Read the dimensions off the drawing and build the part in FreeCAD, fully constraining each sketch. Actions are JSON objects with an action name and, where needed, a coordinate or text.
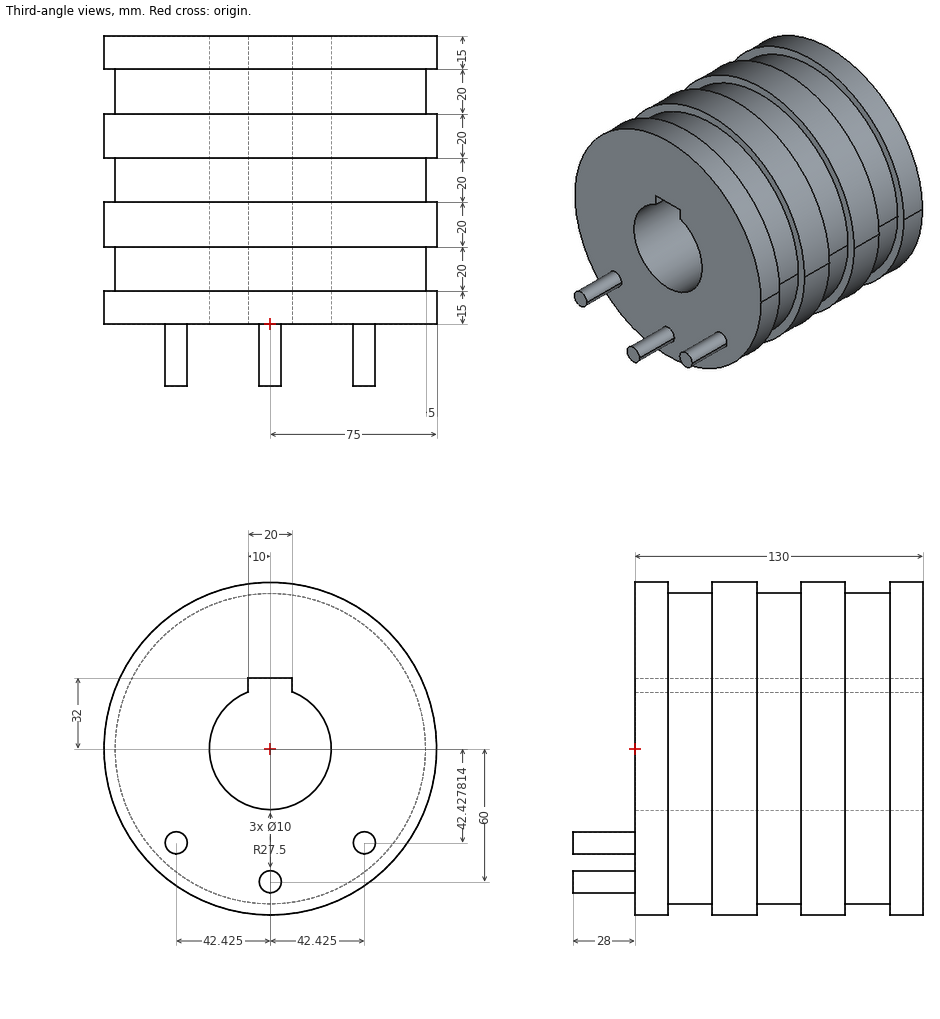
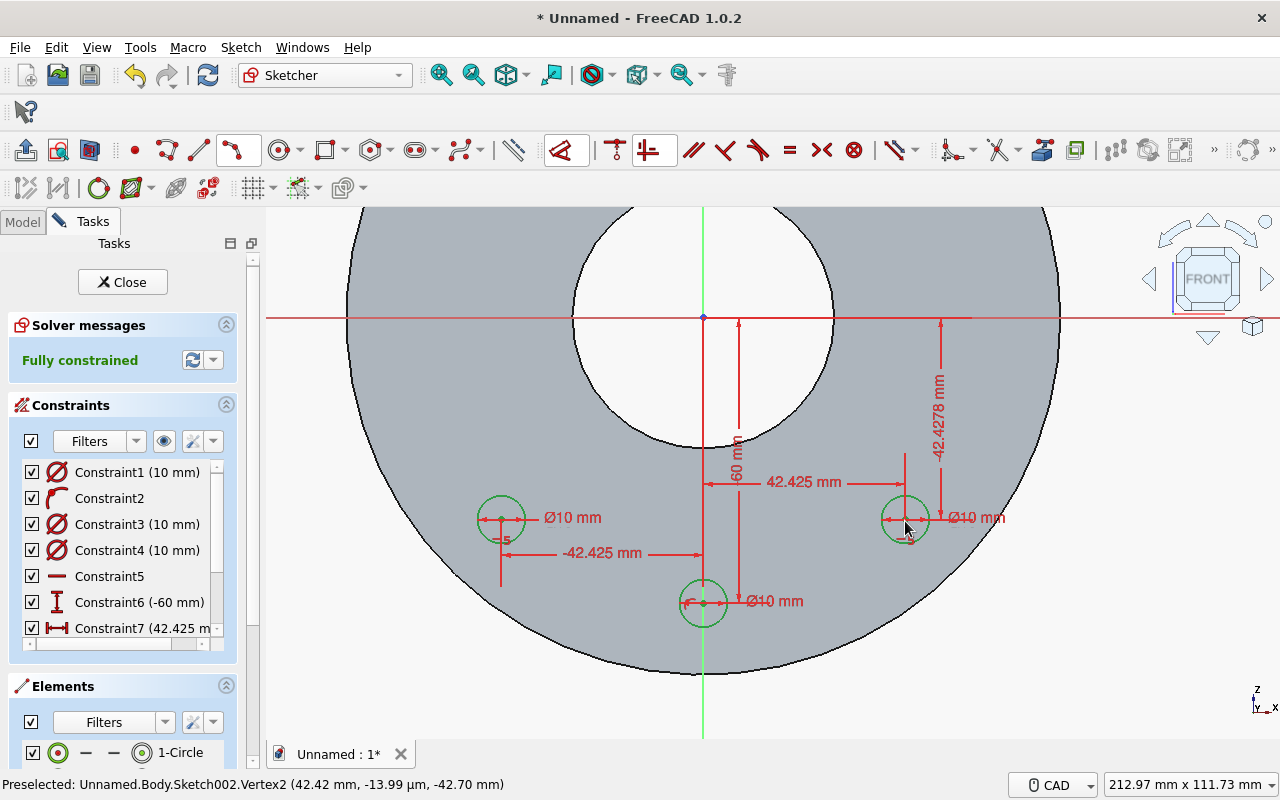
{"action": "left_click", "coordinate": [123, 282]}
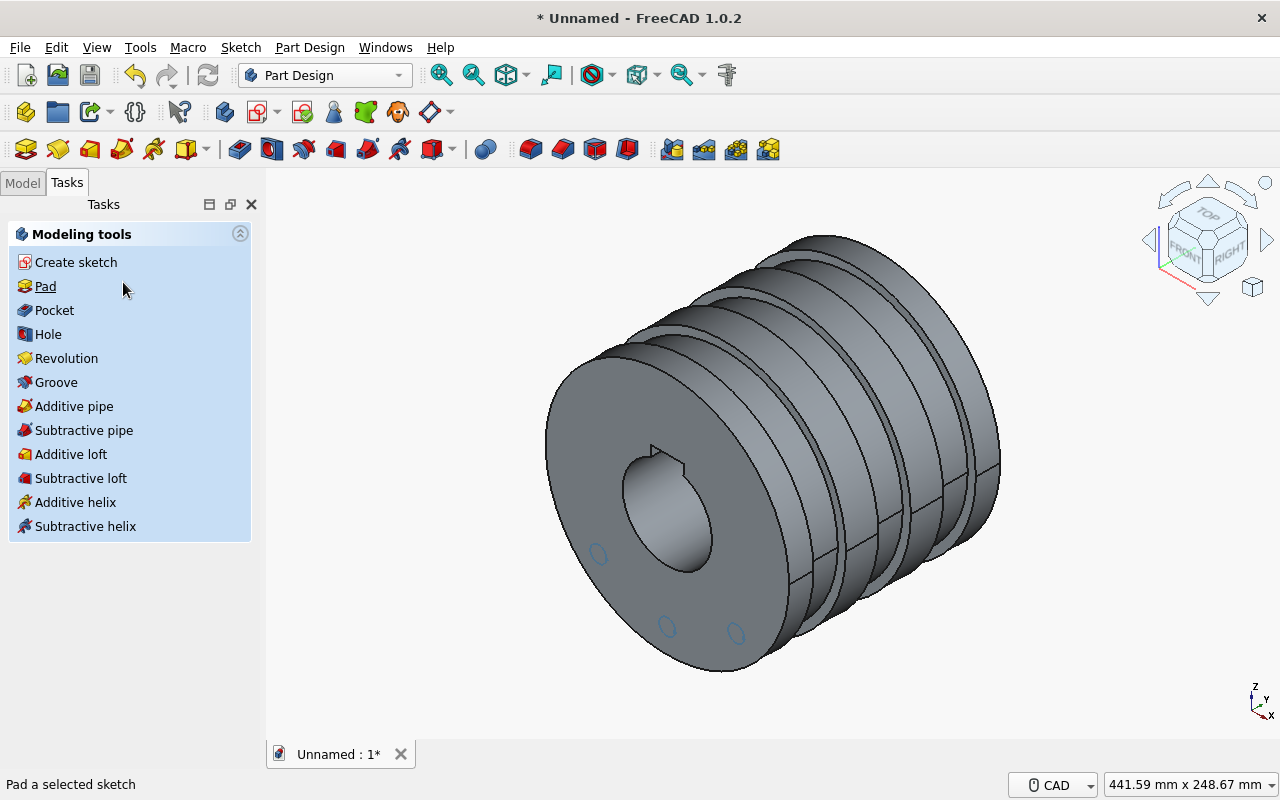
{"action": "left_click", "coordinate": [26, 150]}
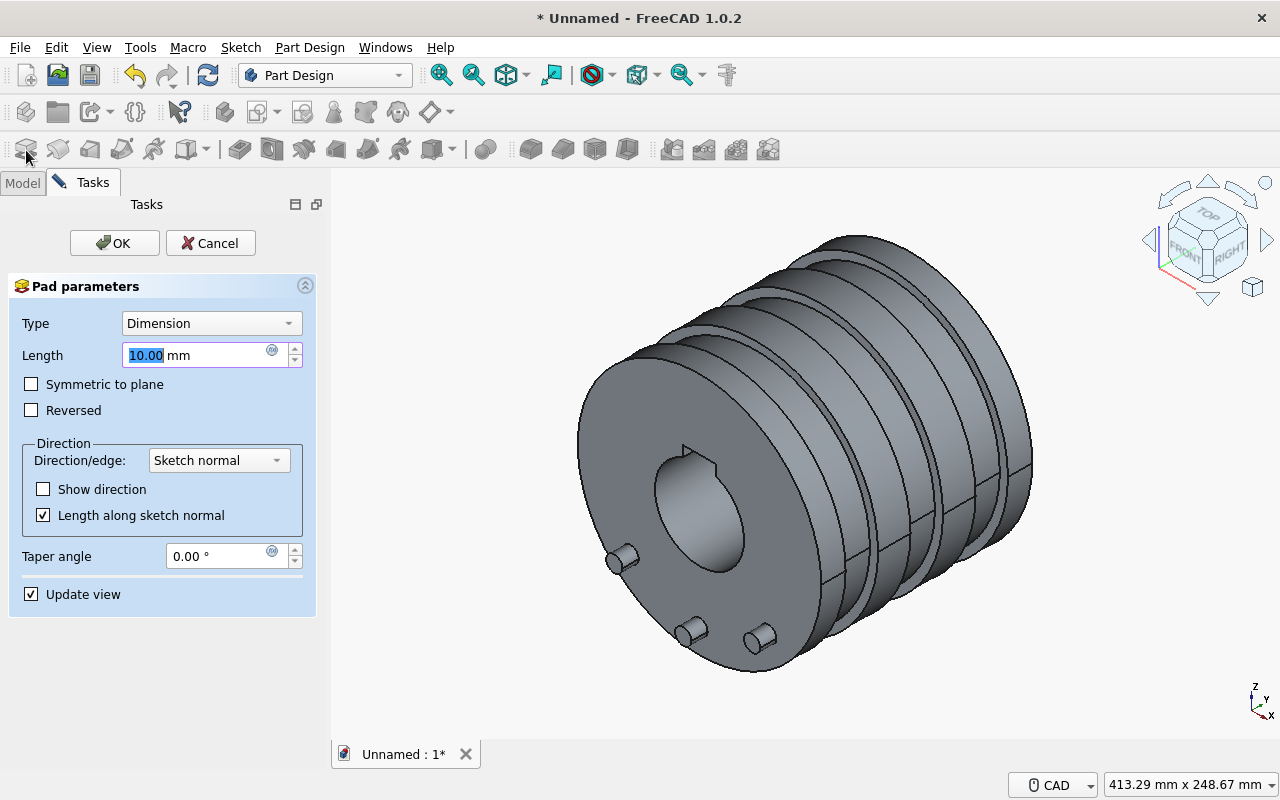
{"action": "type", "text": "28"}
{"action": "key", "text": "Tab"}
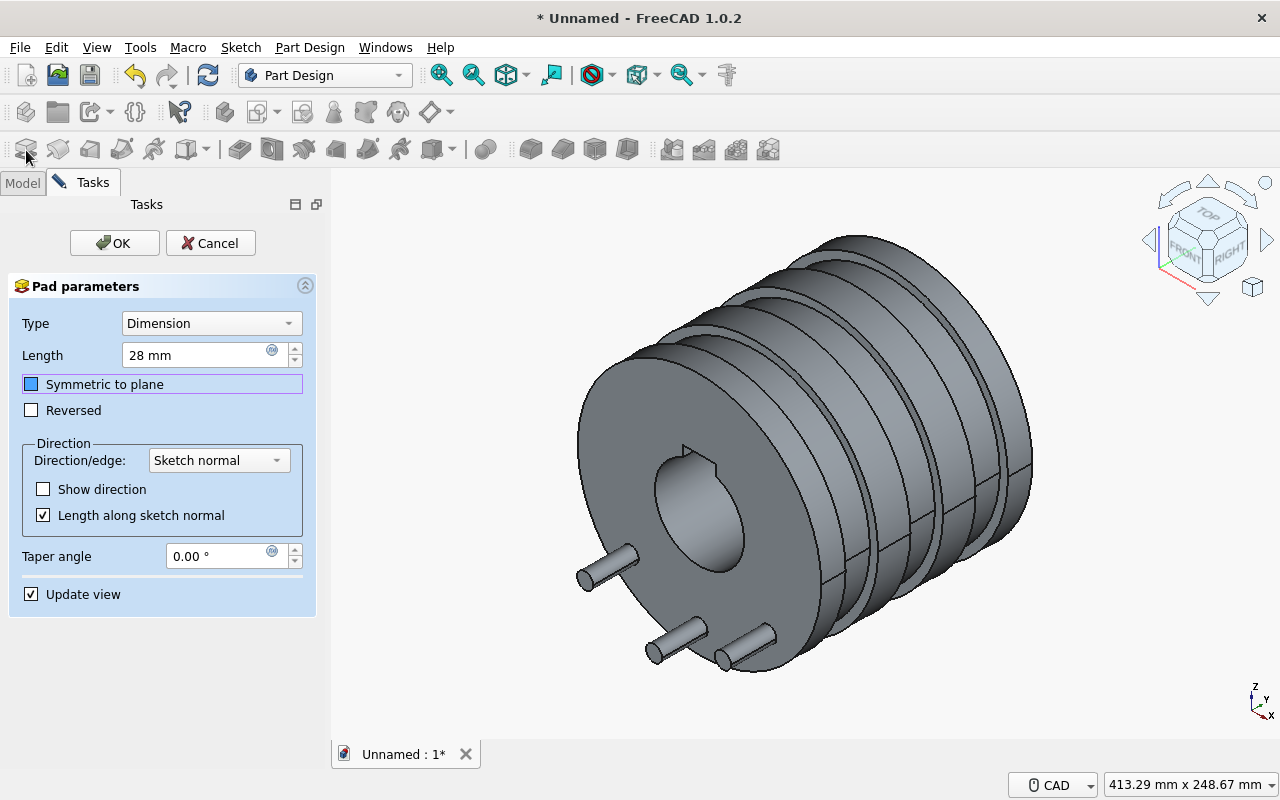
{"action": "left_click", "coordinate": [115, 243]}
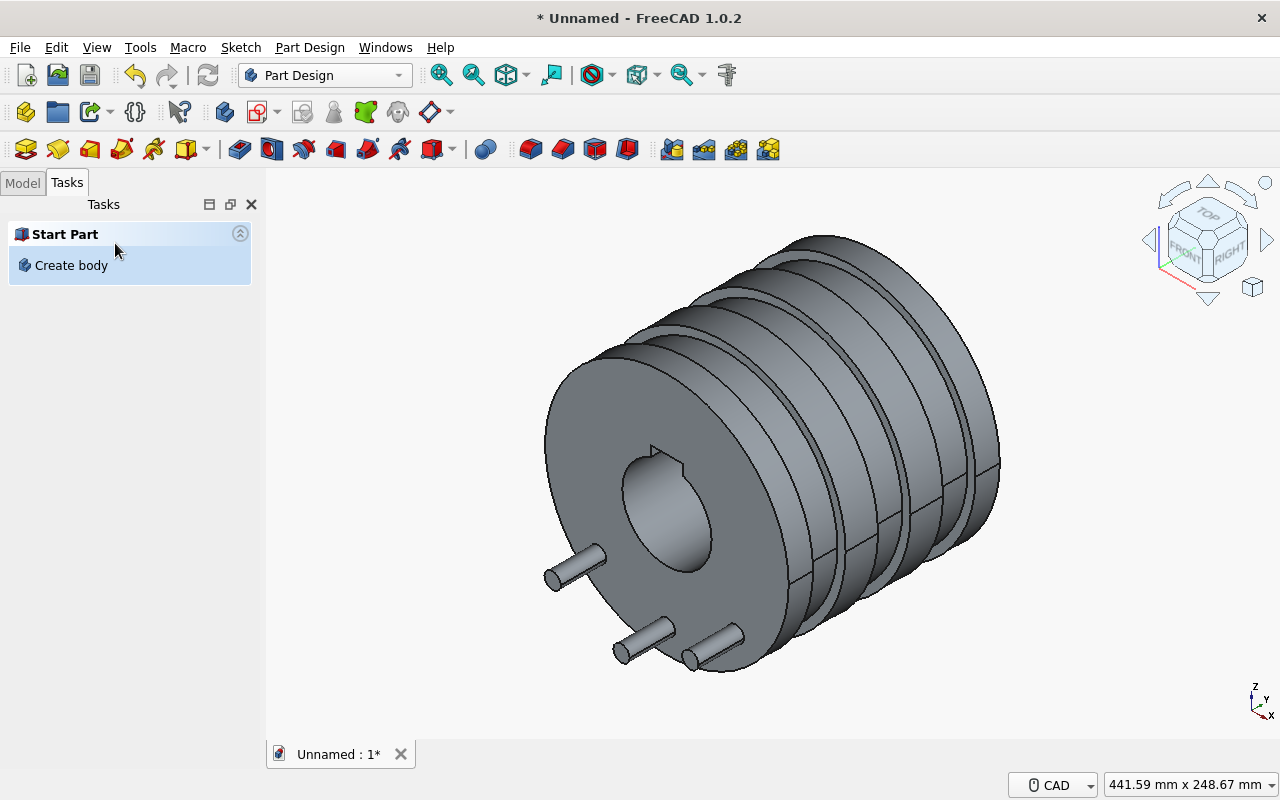
{"action": "key", "text": "v f"}